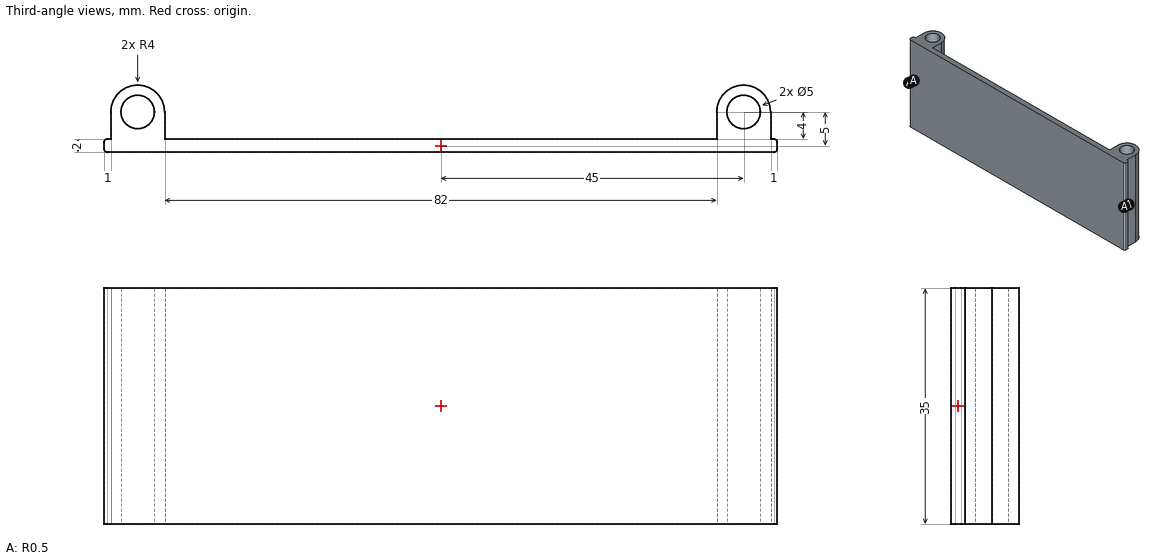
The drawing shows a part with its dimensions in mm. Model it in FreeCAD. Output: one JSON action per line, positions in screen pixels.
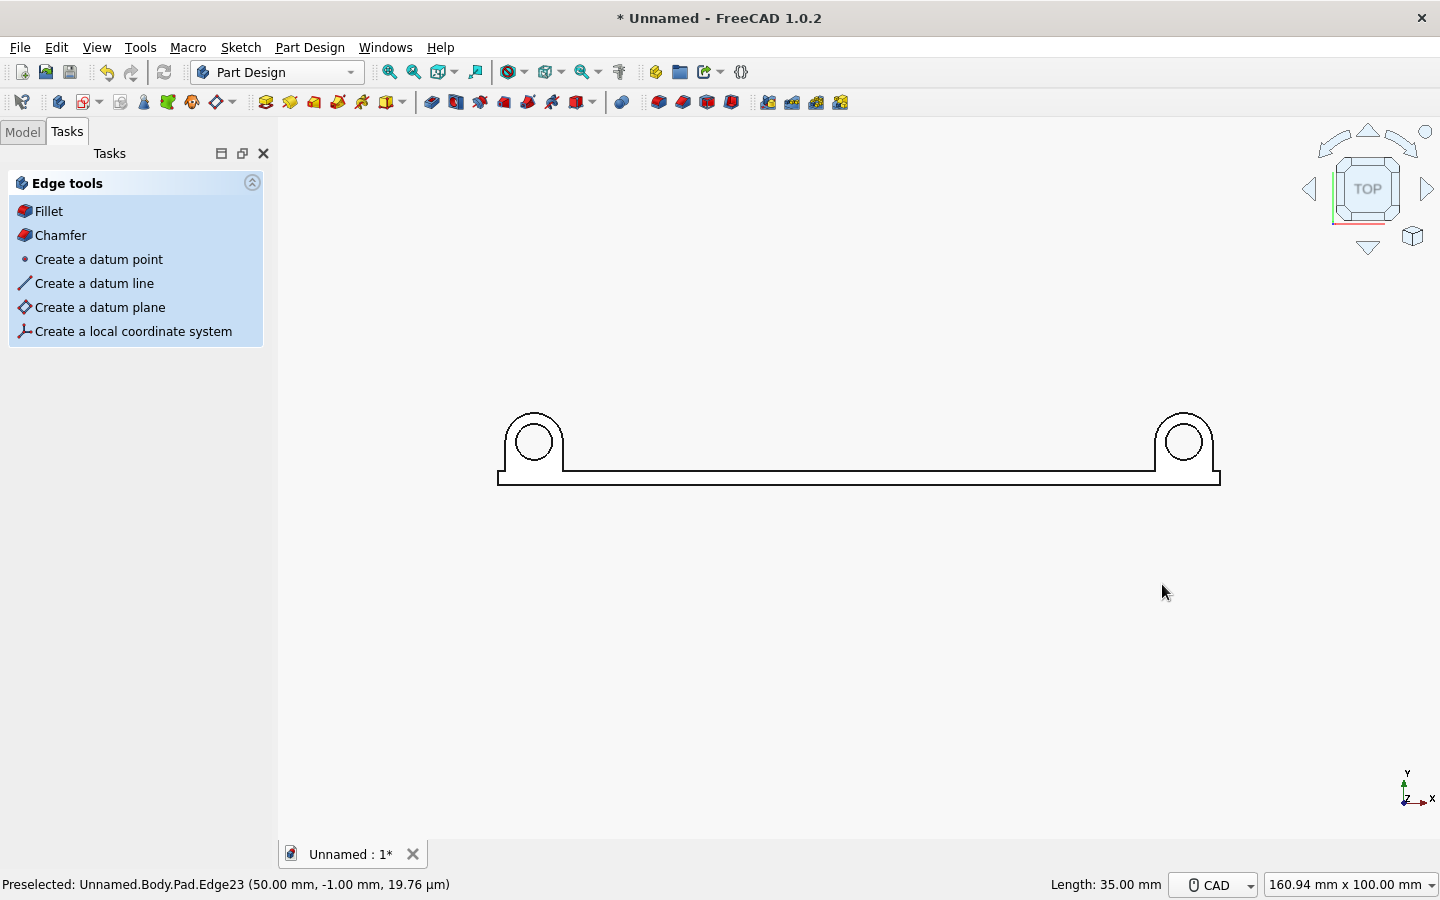
{"action": "key", "text": "1"}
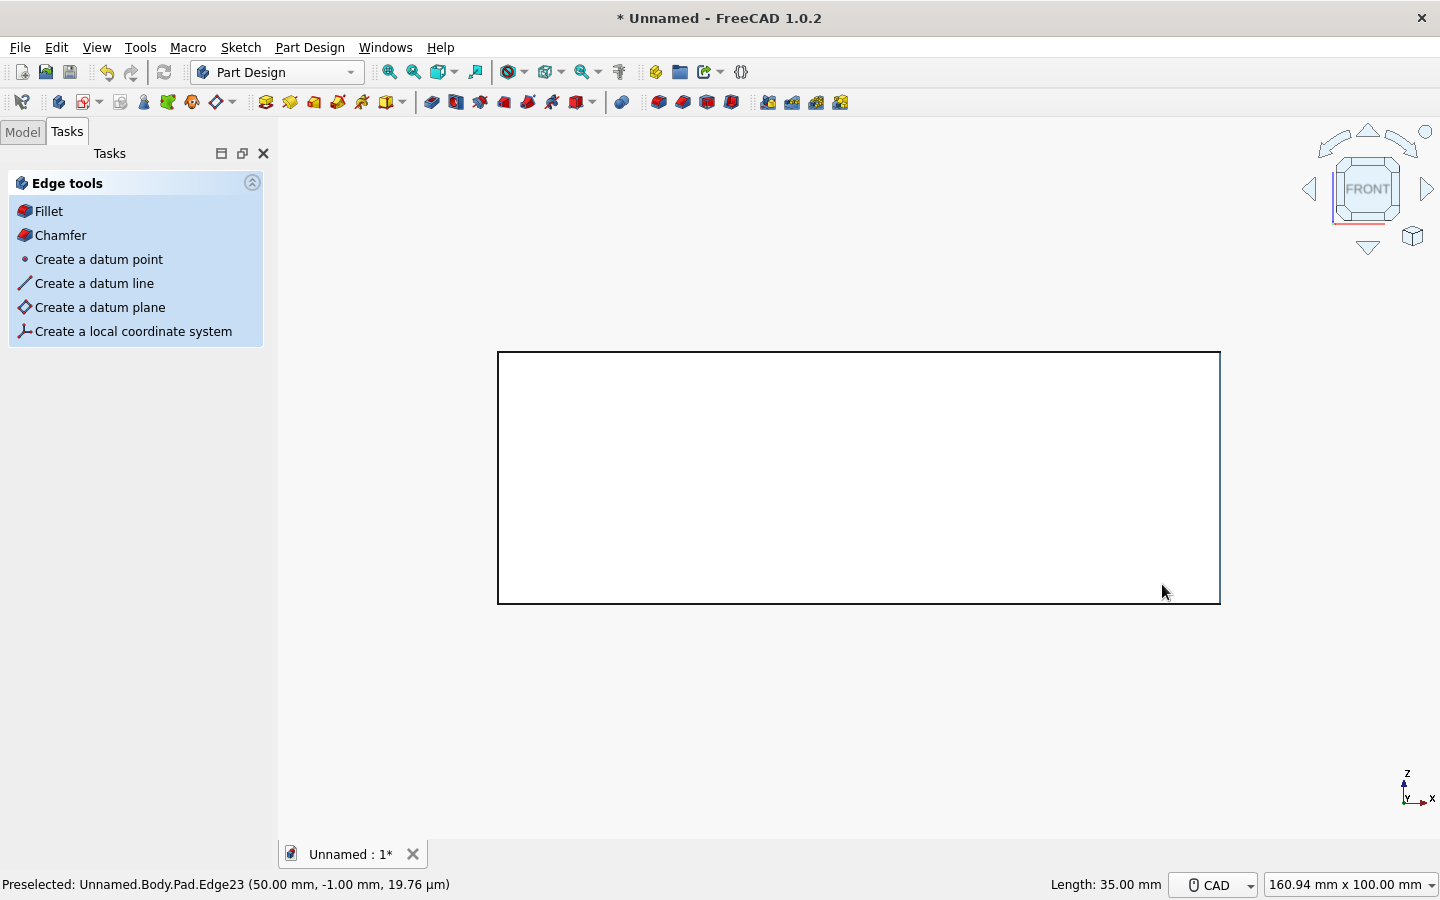
{"action": "left_click", "coordinate": [498, 477], "text": "ctrl"}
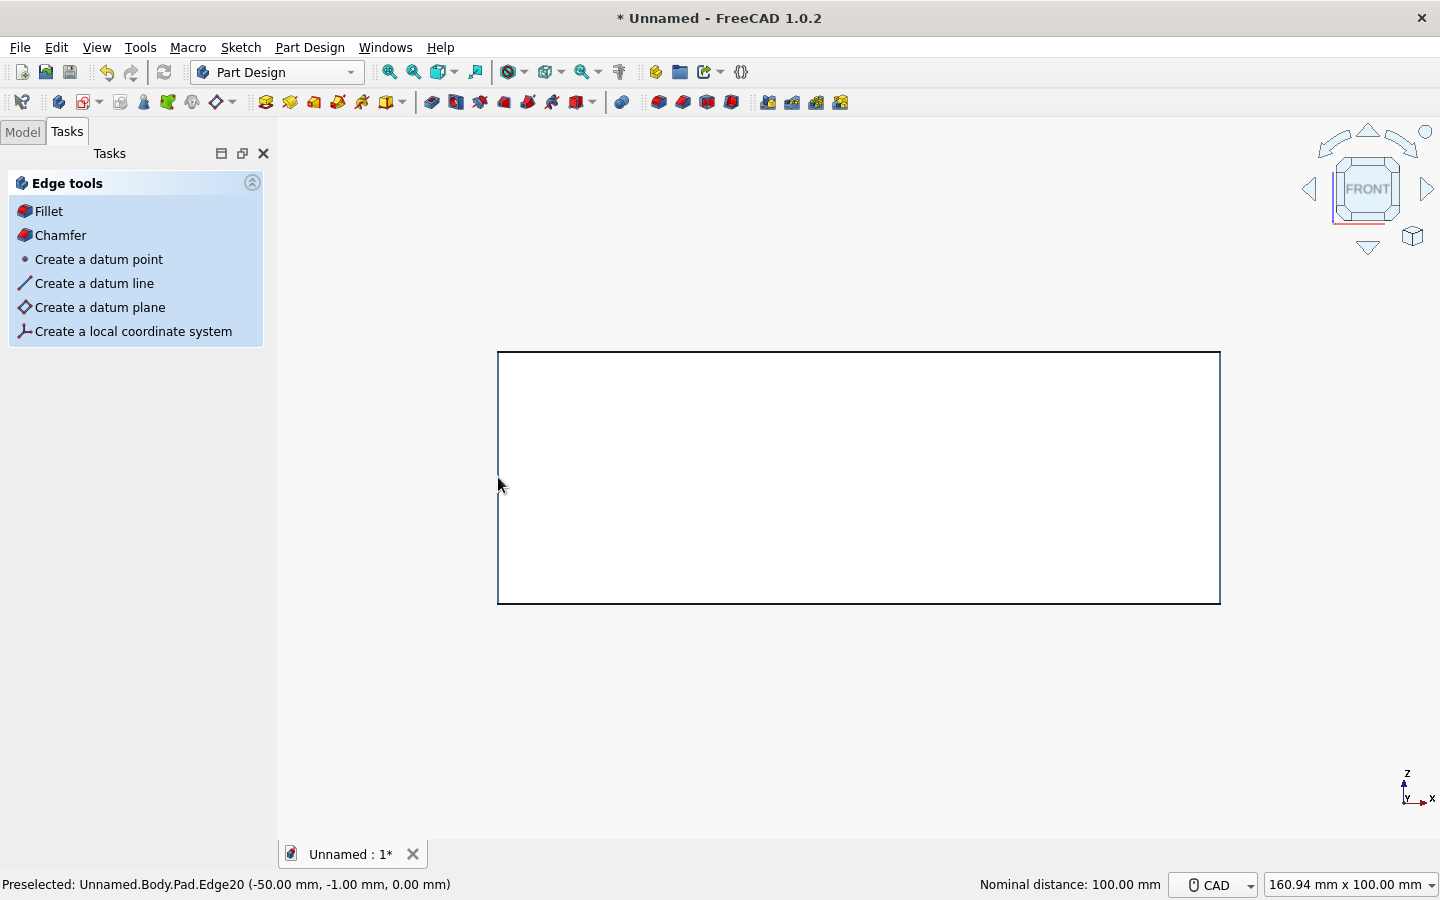
{"action": "key", "text": "3"}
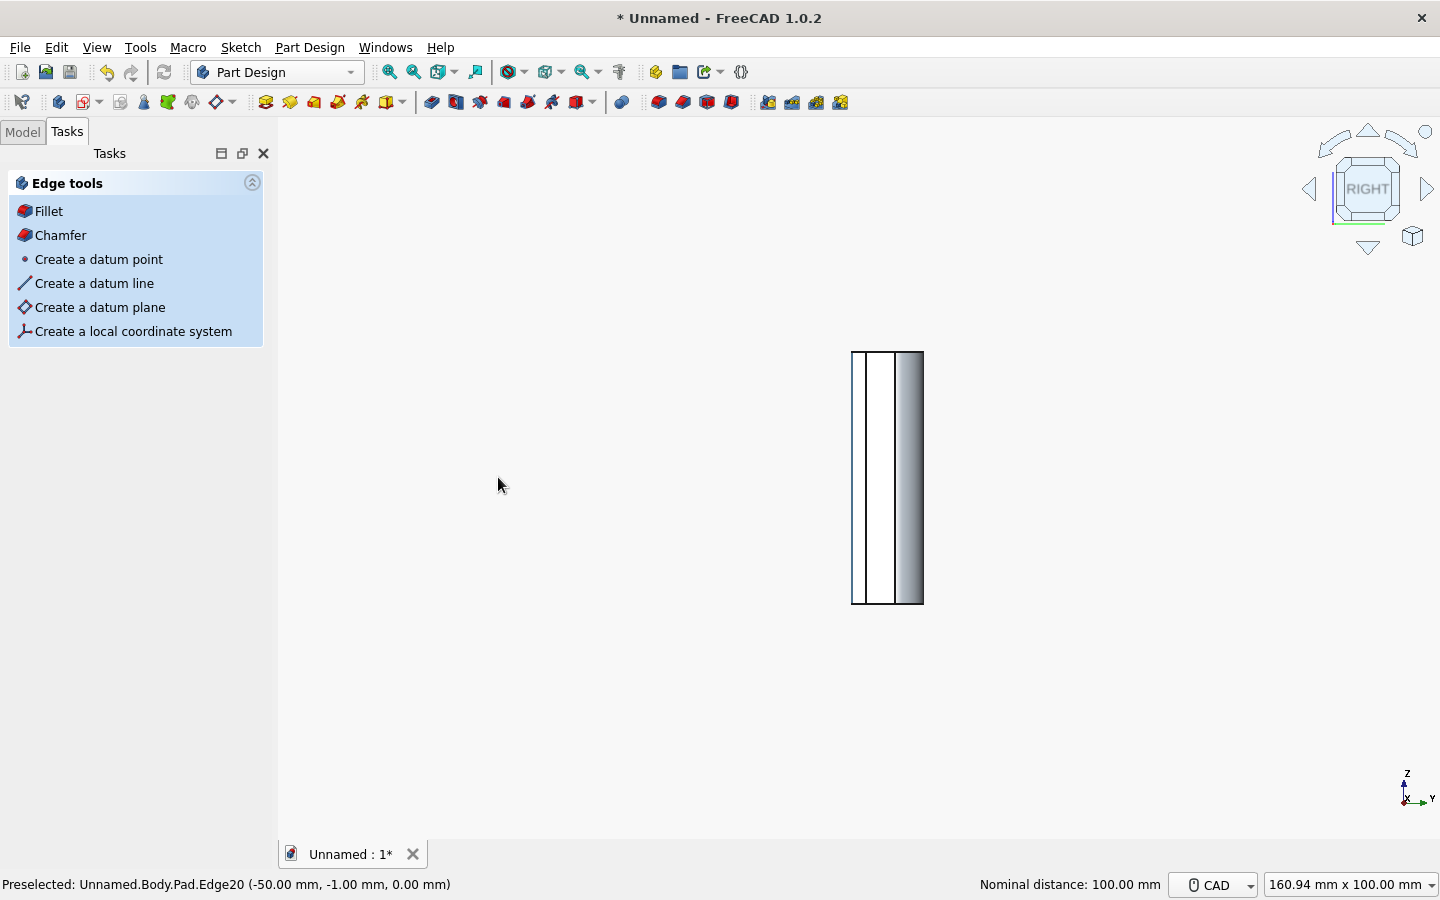
{"action": "left_click", "coordinate": [390, 72]}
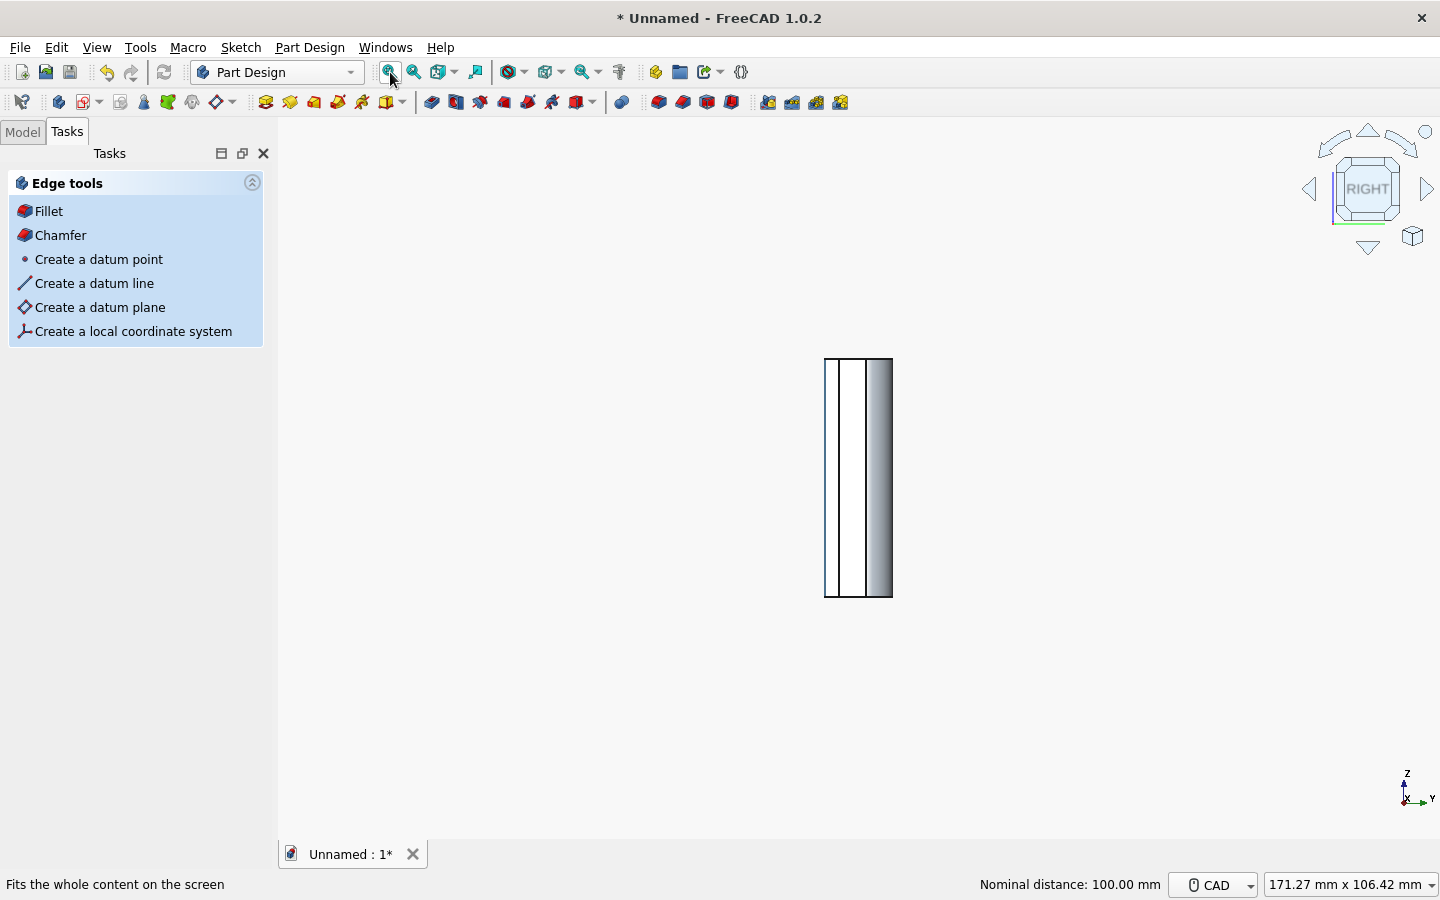
{"action": "left_click", "coordinate": [839, 477], "text": "ctrl"}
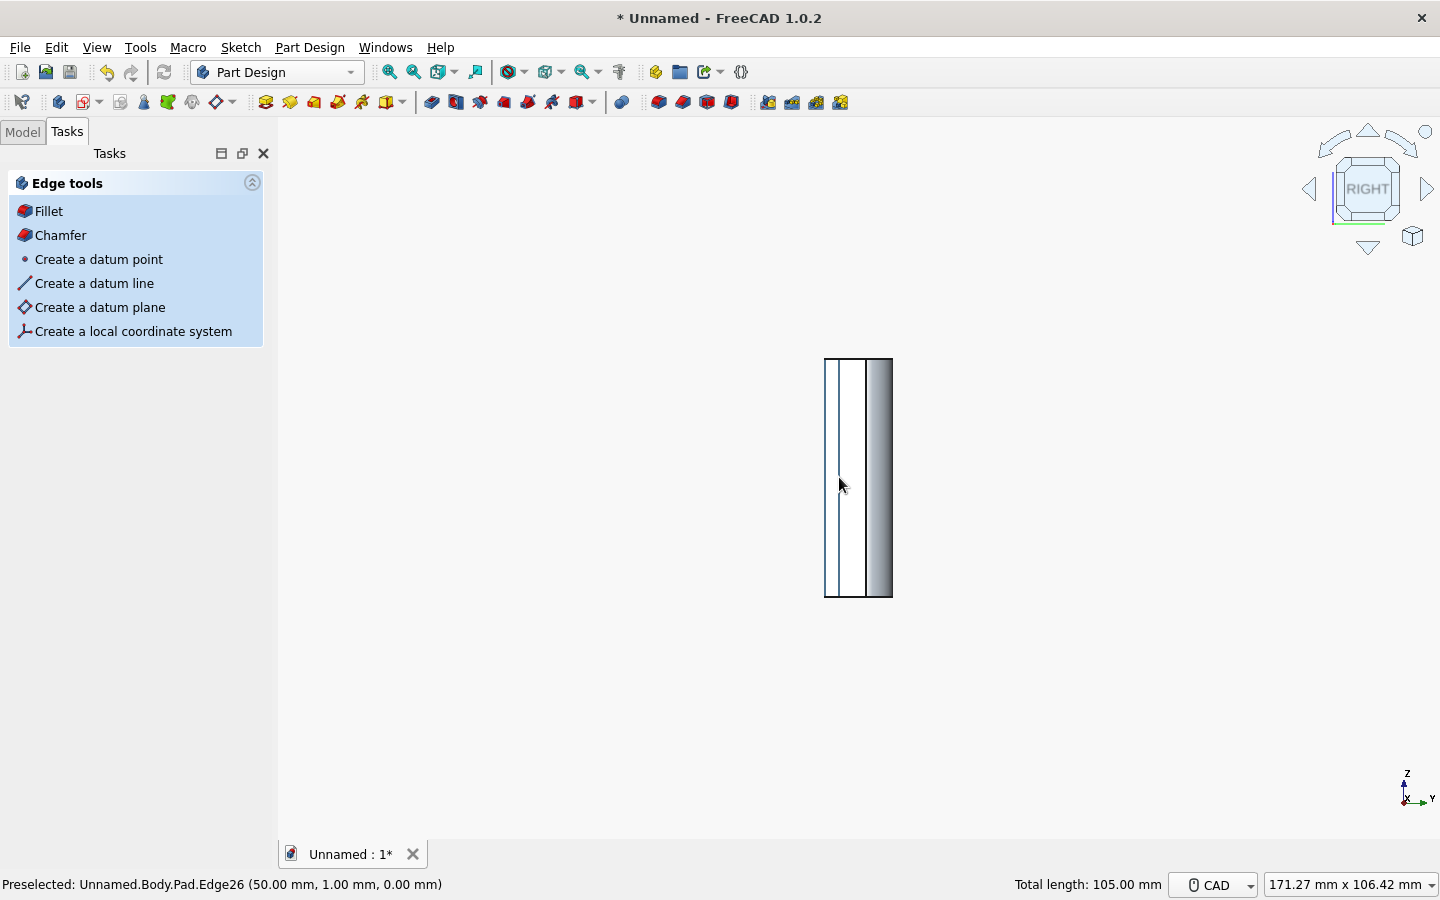
{"action": "key", "text": "5"}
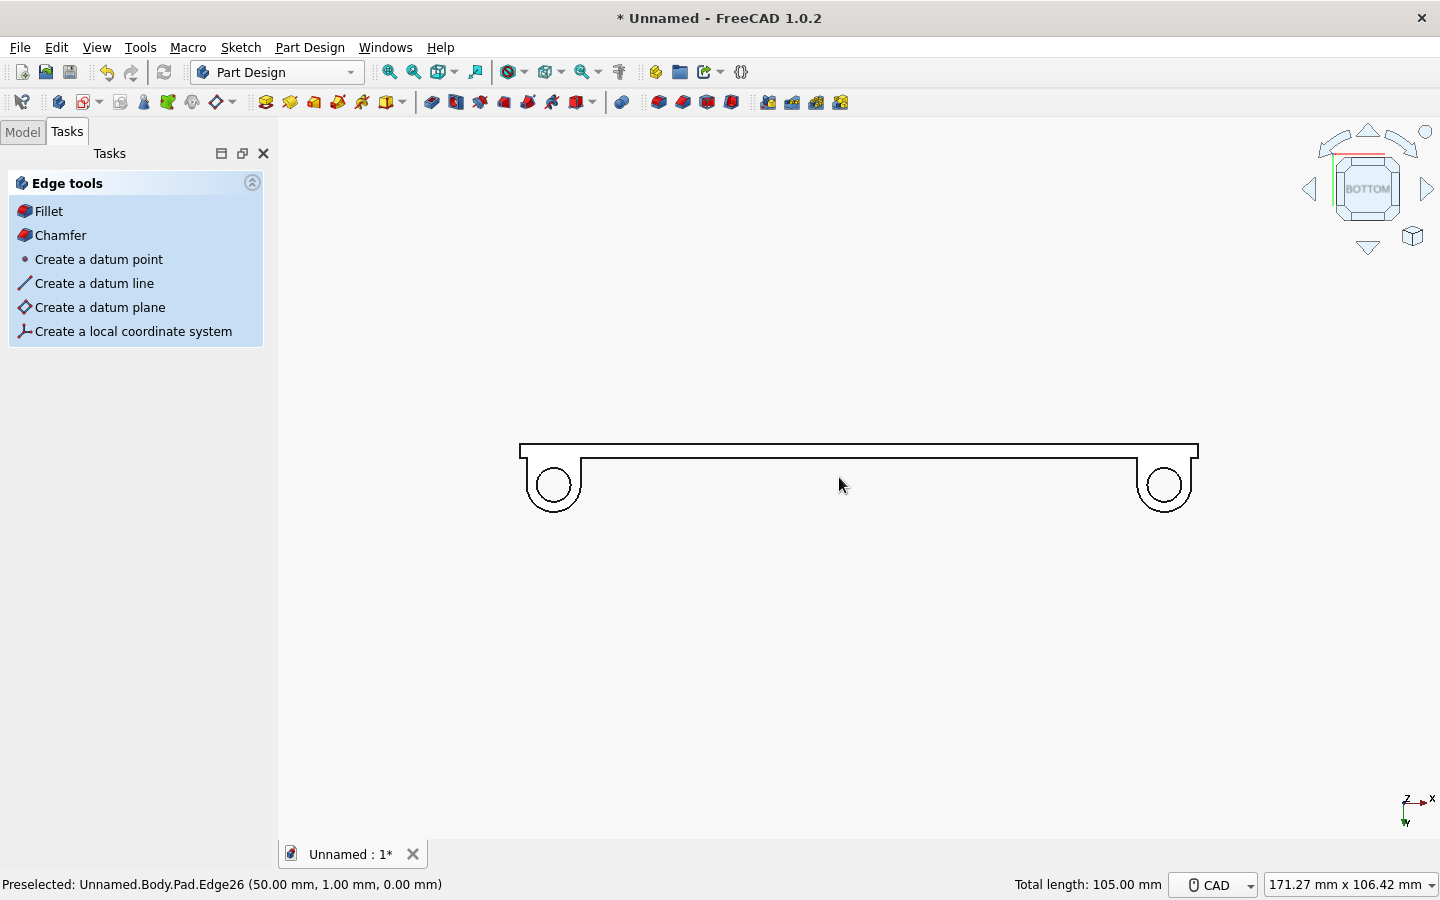
{"action": "key", "text": "4"}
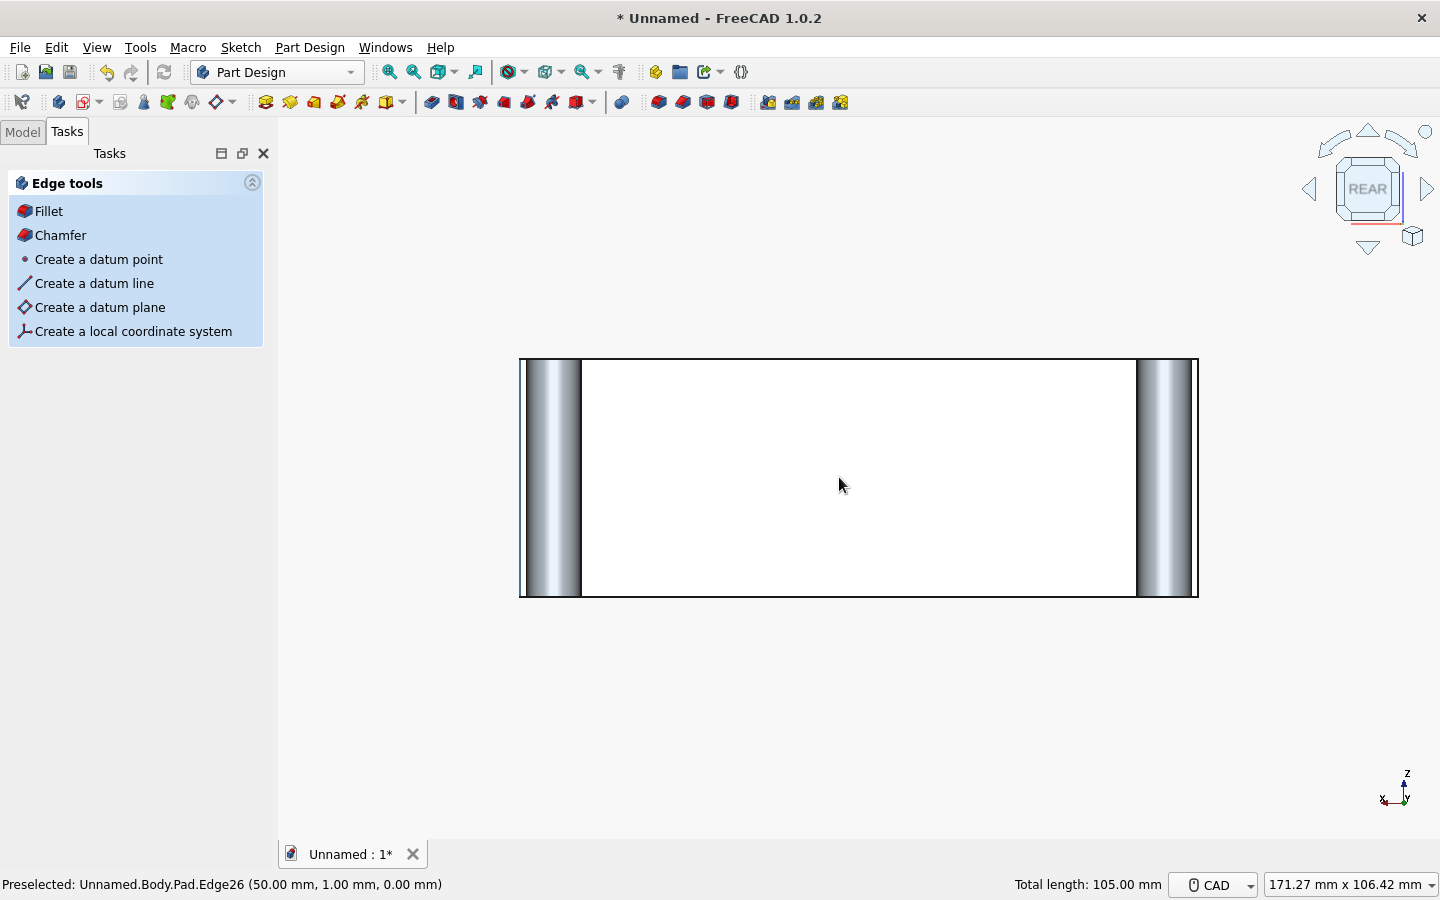
{"action": "left_click", "coordinate": [1198, 477], "text": "ctrl"}